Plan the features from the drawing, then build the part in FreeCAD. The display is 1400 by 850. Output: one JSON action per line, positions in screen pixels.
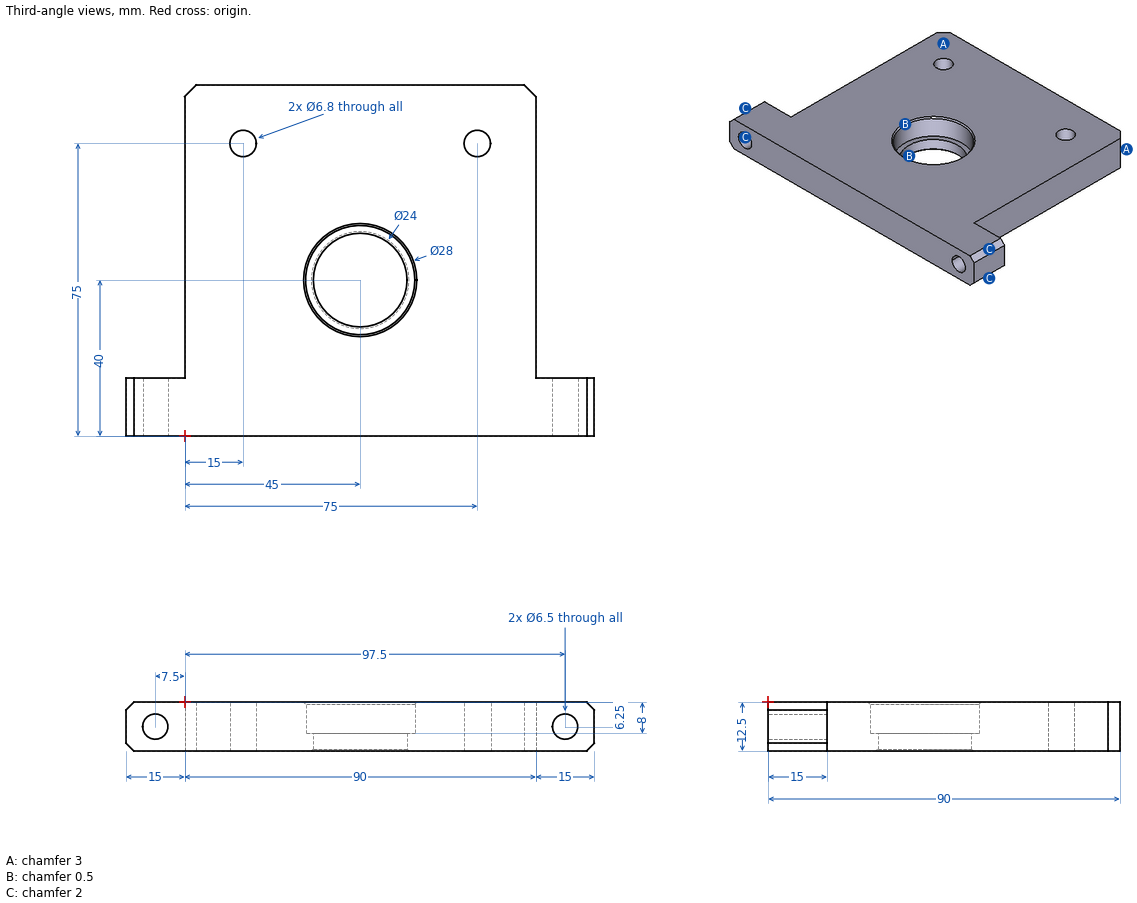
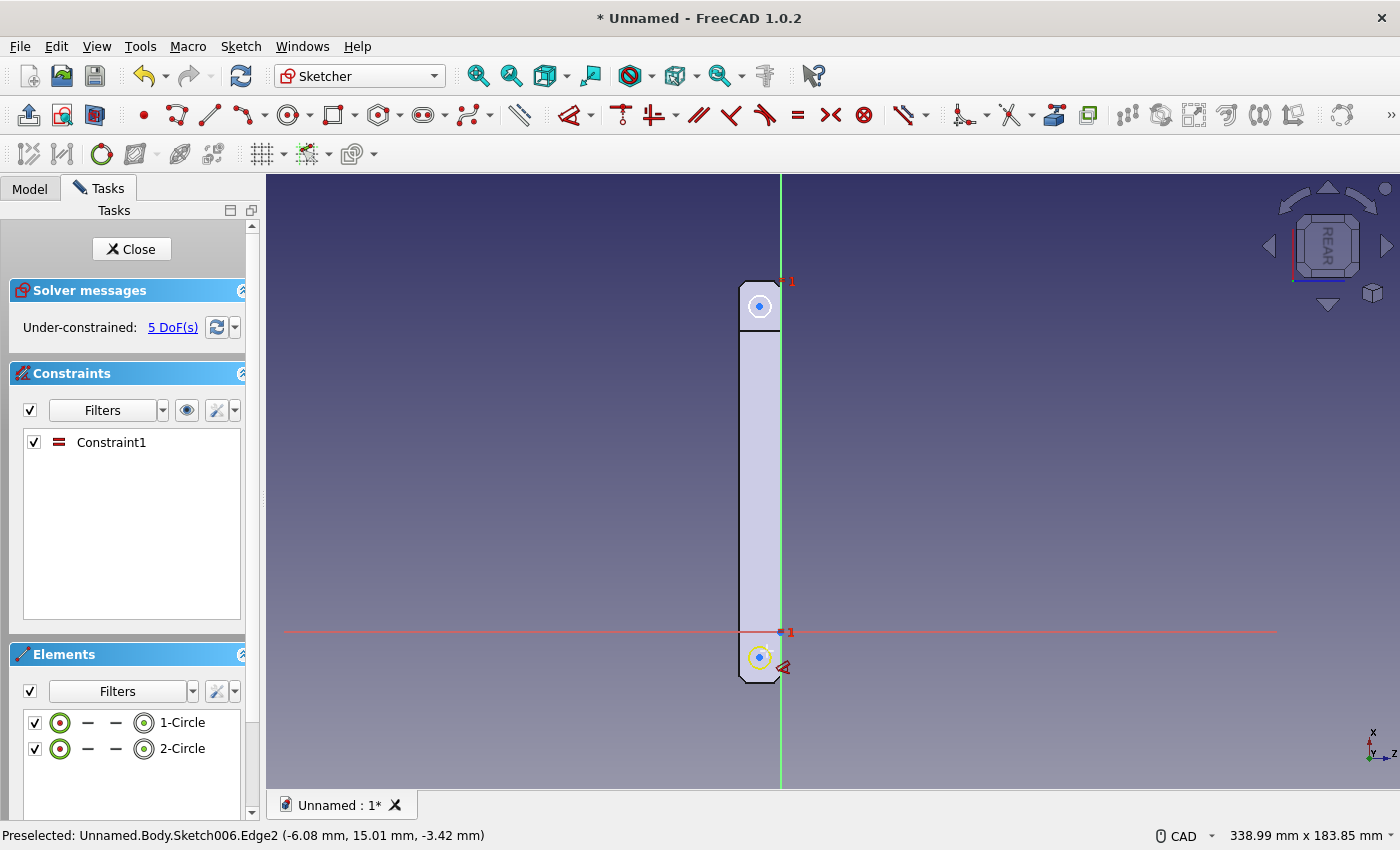
{"action": "scroll", "coordinate": [768, 299], "scroll_direction": "up", "scroll_amount": 4}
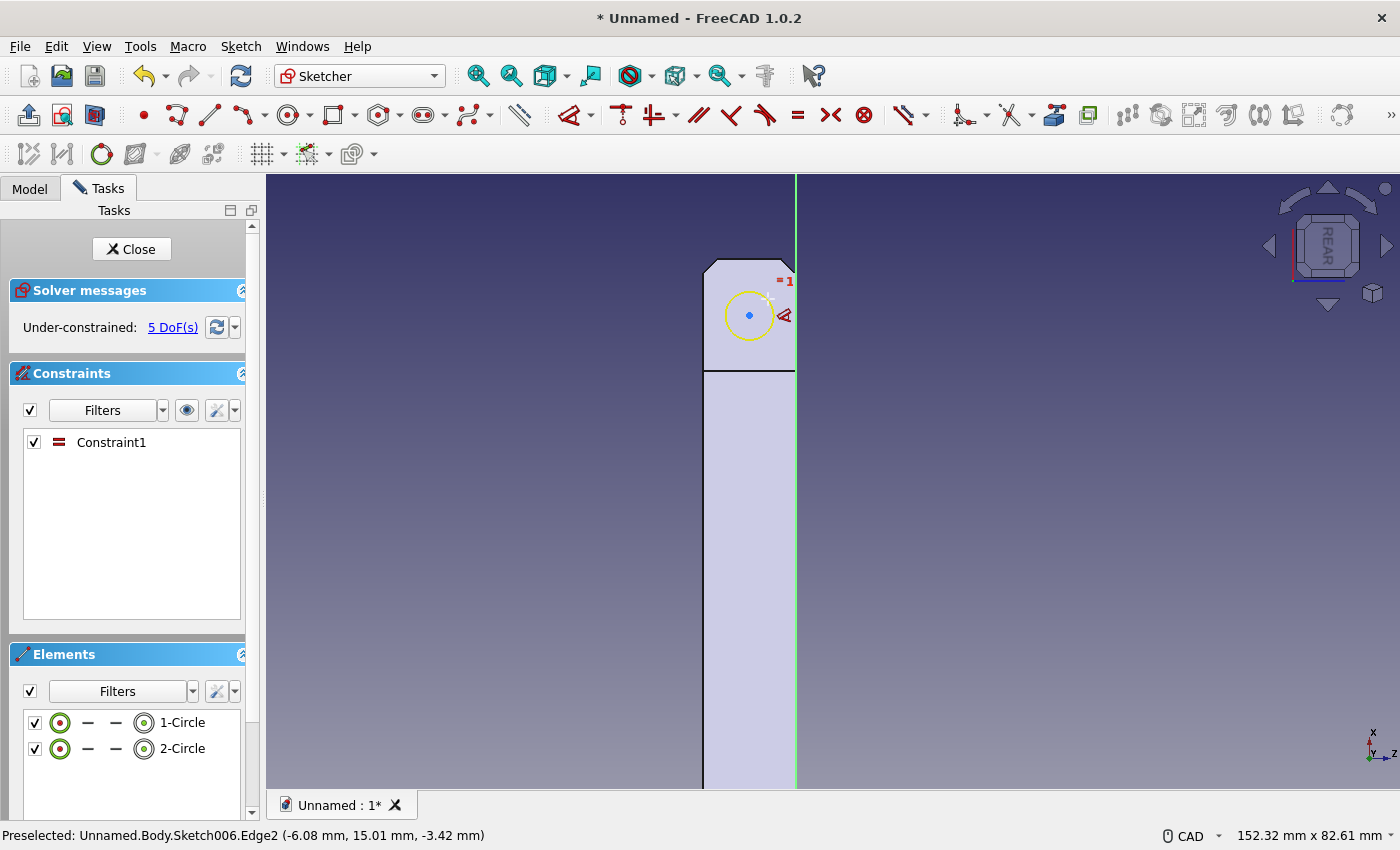
{"action": "left_click", "coordinate": [767, 299]}
{"action": "left_click", "coordinate": [766, 262]}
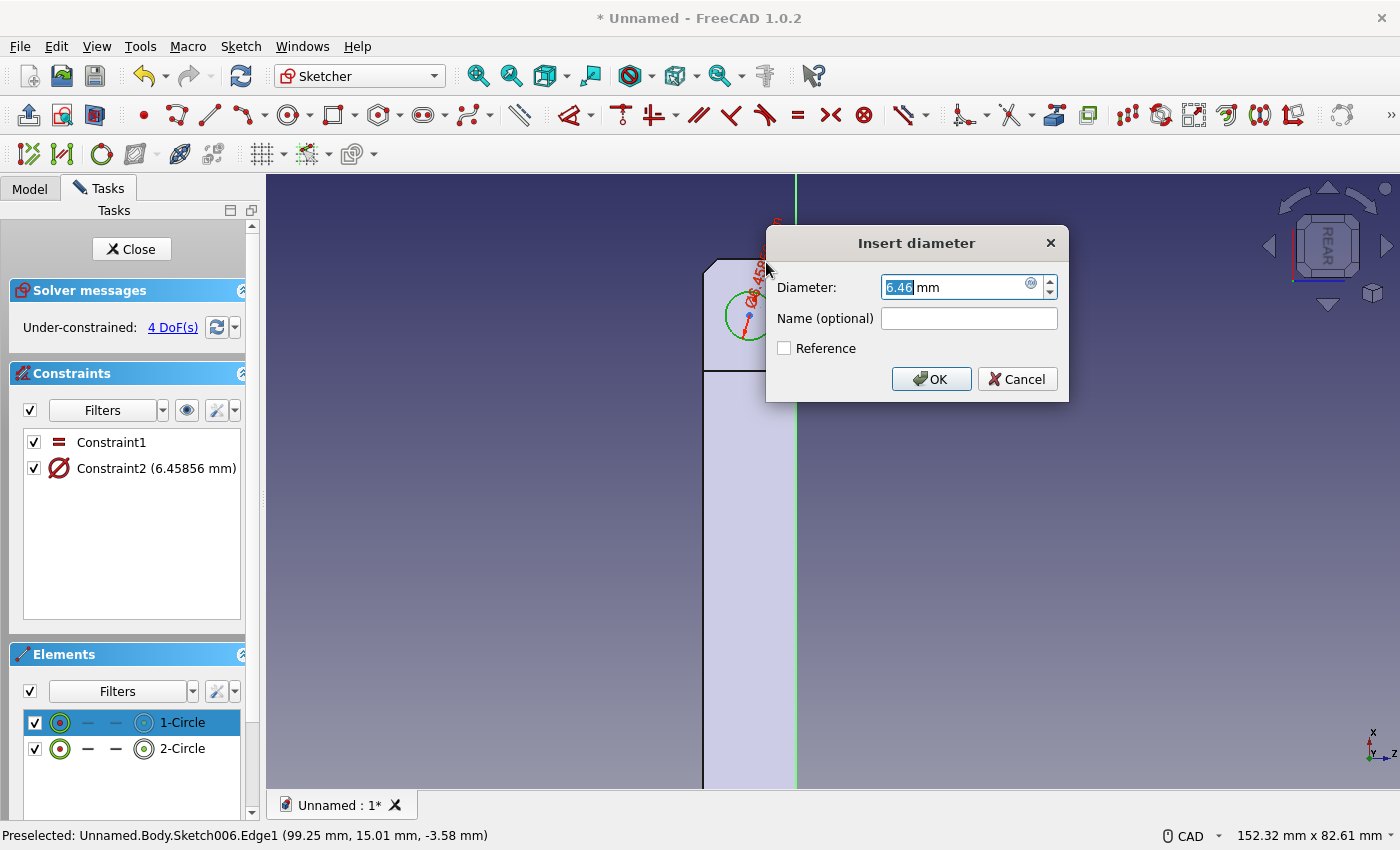
{"action": "type", "text": "6.5"}
{"action": "key", "text": "Return"}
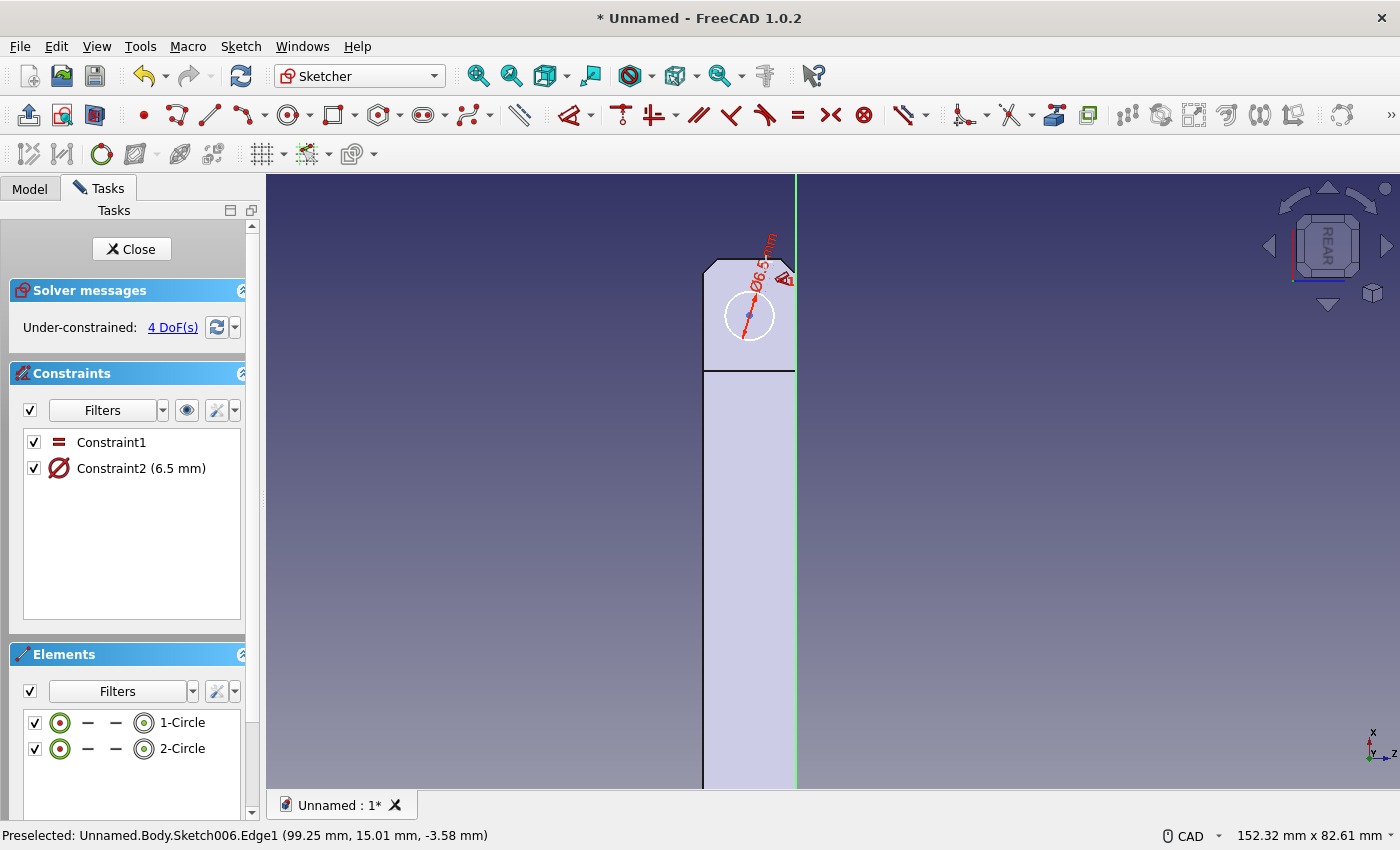
{"action": "scroll", "coordinate": [768, 299], "scroll_direction": "down", "scroll_amount": 4}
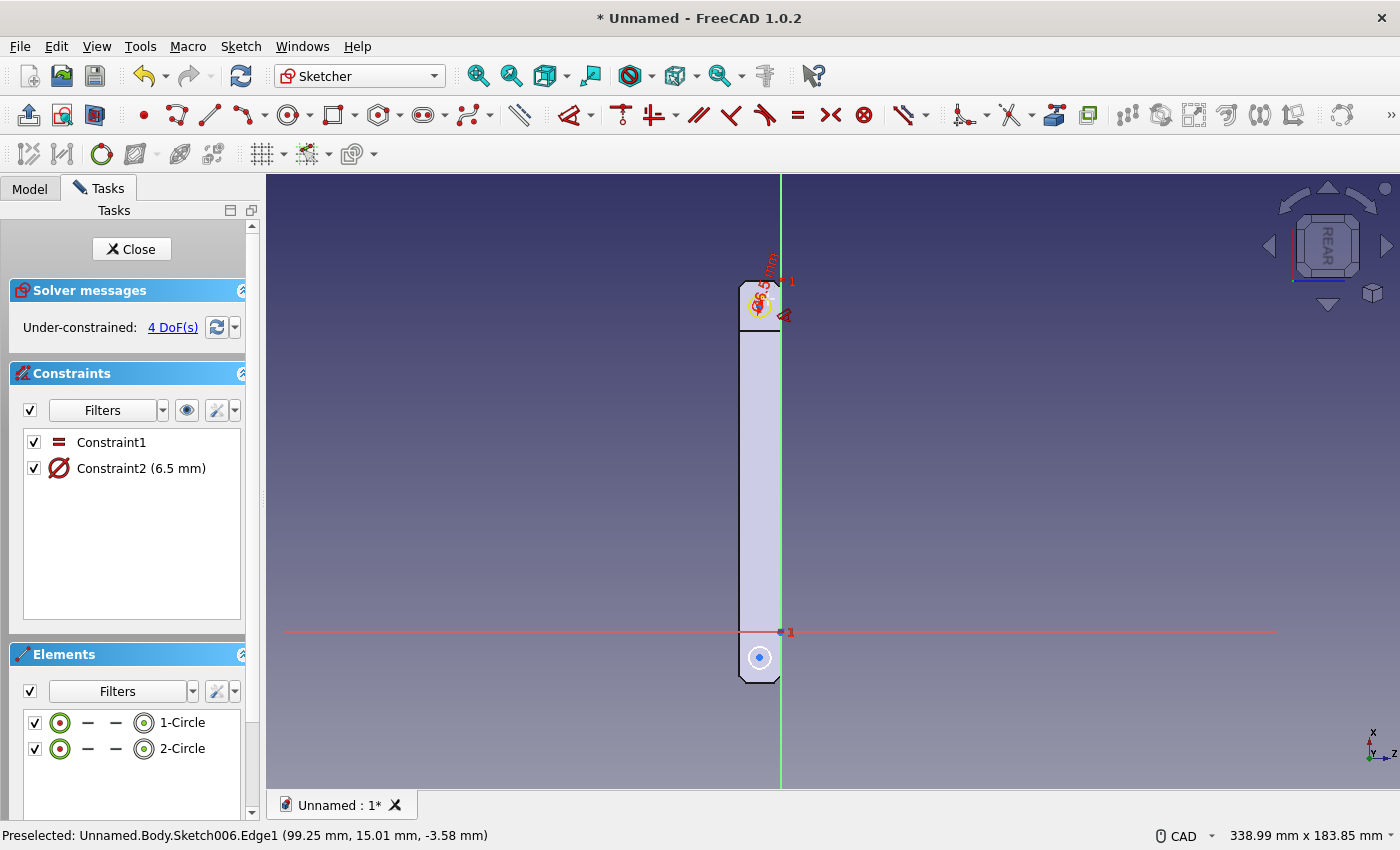
{"action": "scroll", "coordinate": [760, 658], "scroll_direction": "up", "scroll_amount": 3}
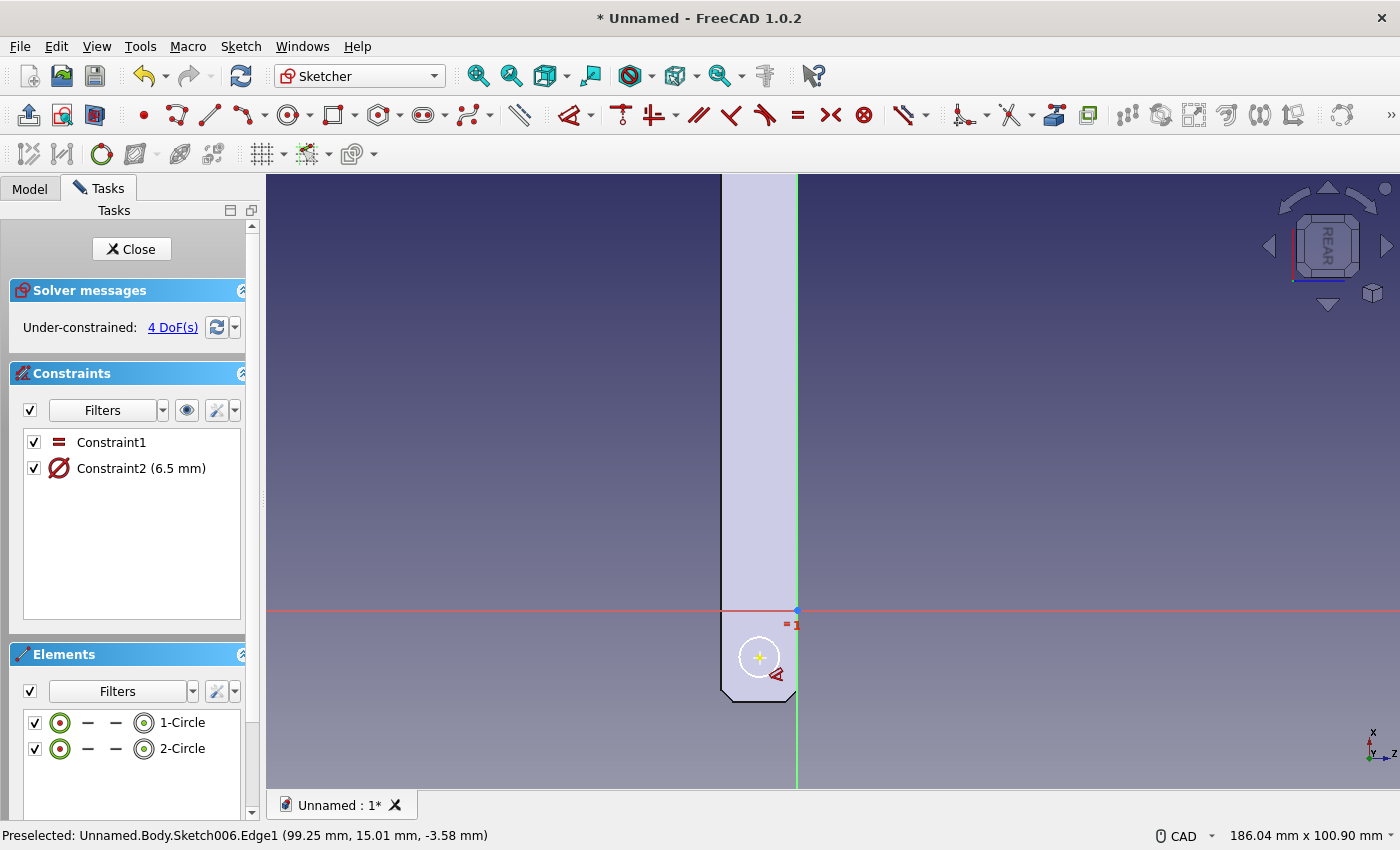
{"action": "left_click", "coordinate": [759, 657]}
{"action": "left_click", "coordinate": [831, 634]}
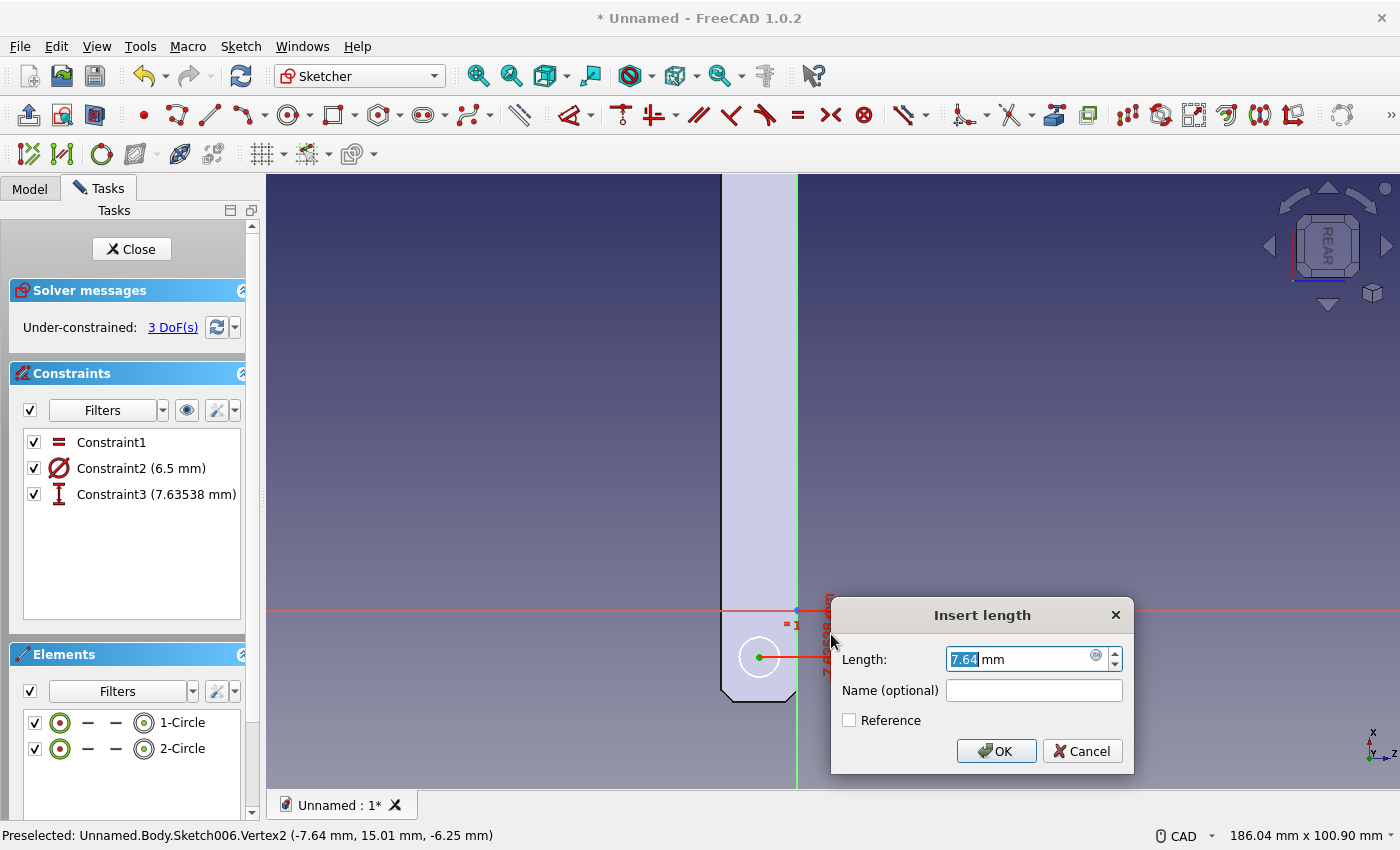
{"action": "type", "text": "7.5"}
{"action": "key", "text": "Return"}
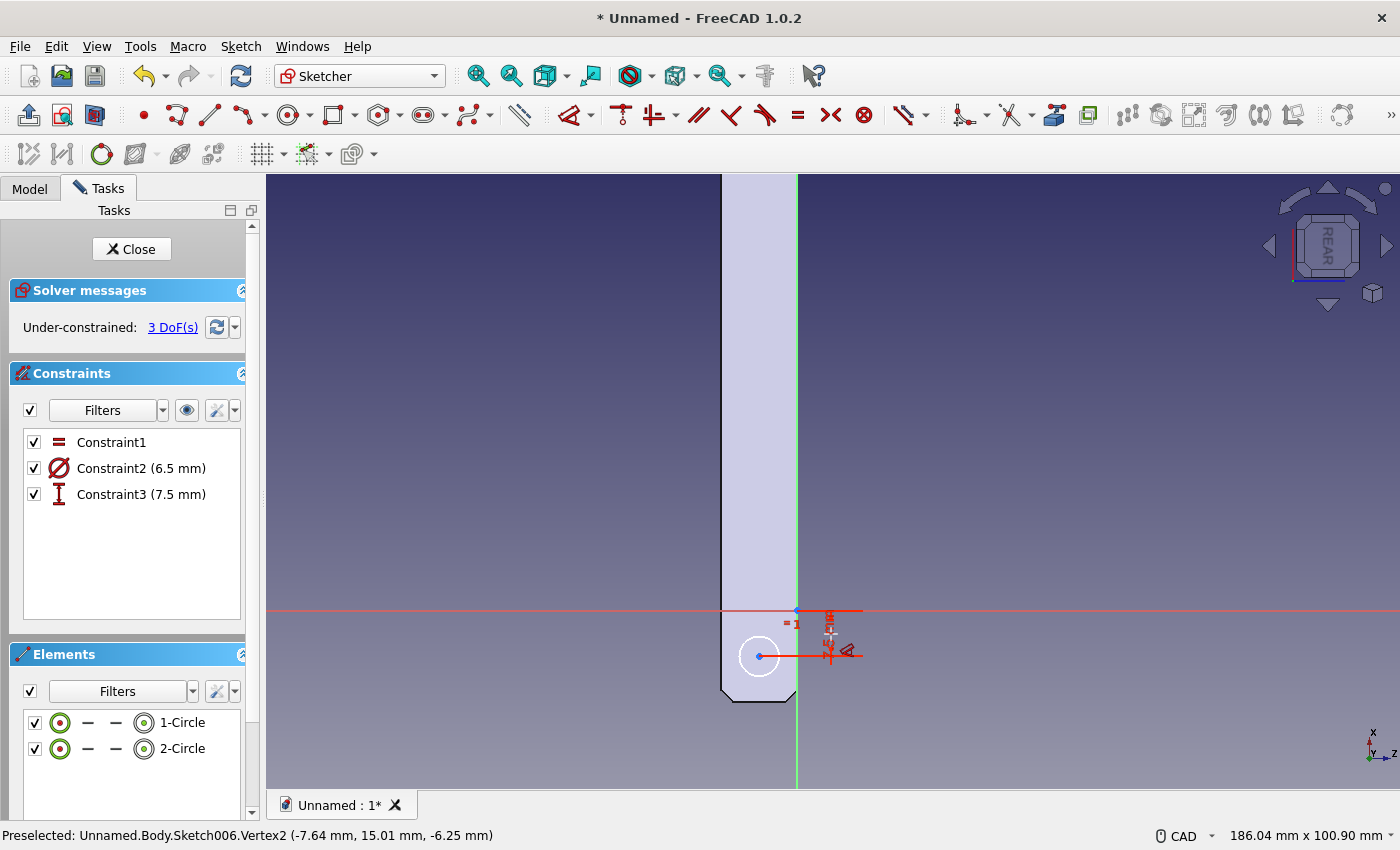
{"action": "scroll", "coordinate": [760, 658], "scroll_direction": "down", "scroll_amount": 3}